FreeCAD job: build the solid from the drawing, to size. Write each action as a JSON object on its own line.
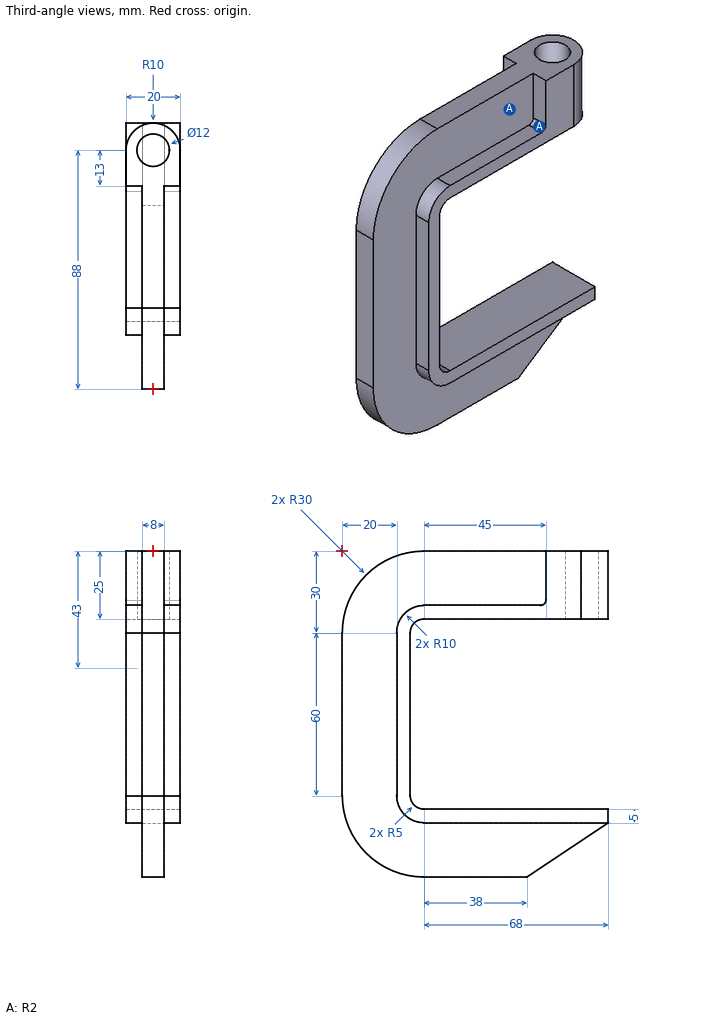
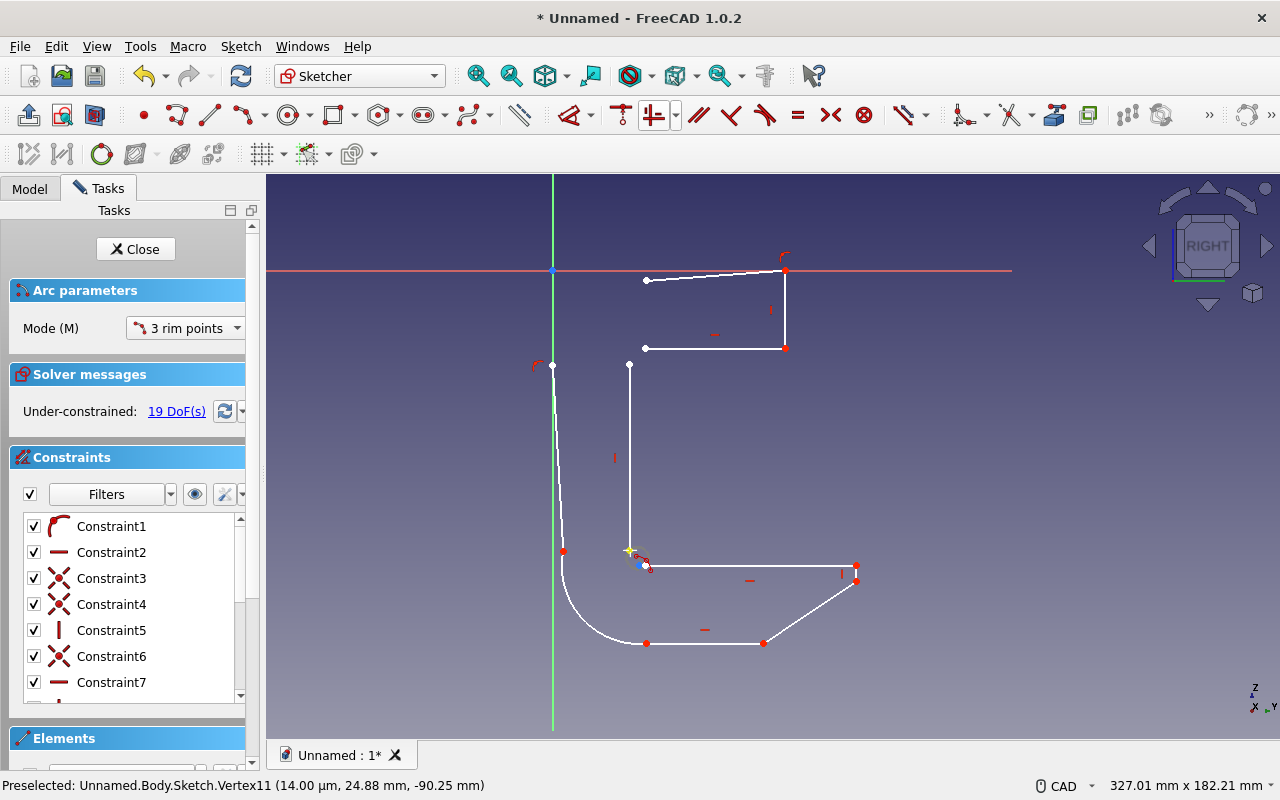
{"action": "scroll", "coordinate": [635, 561], "scroll_direction": "up", "scroll_amount": 7}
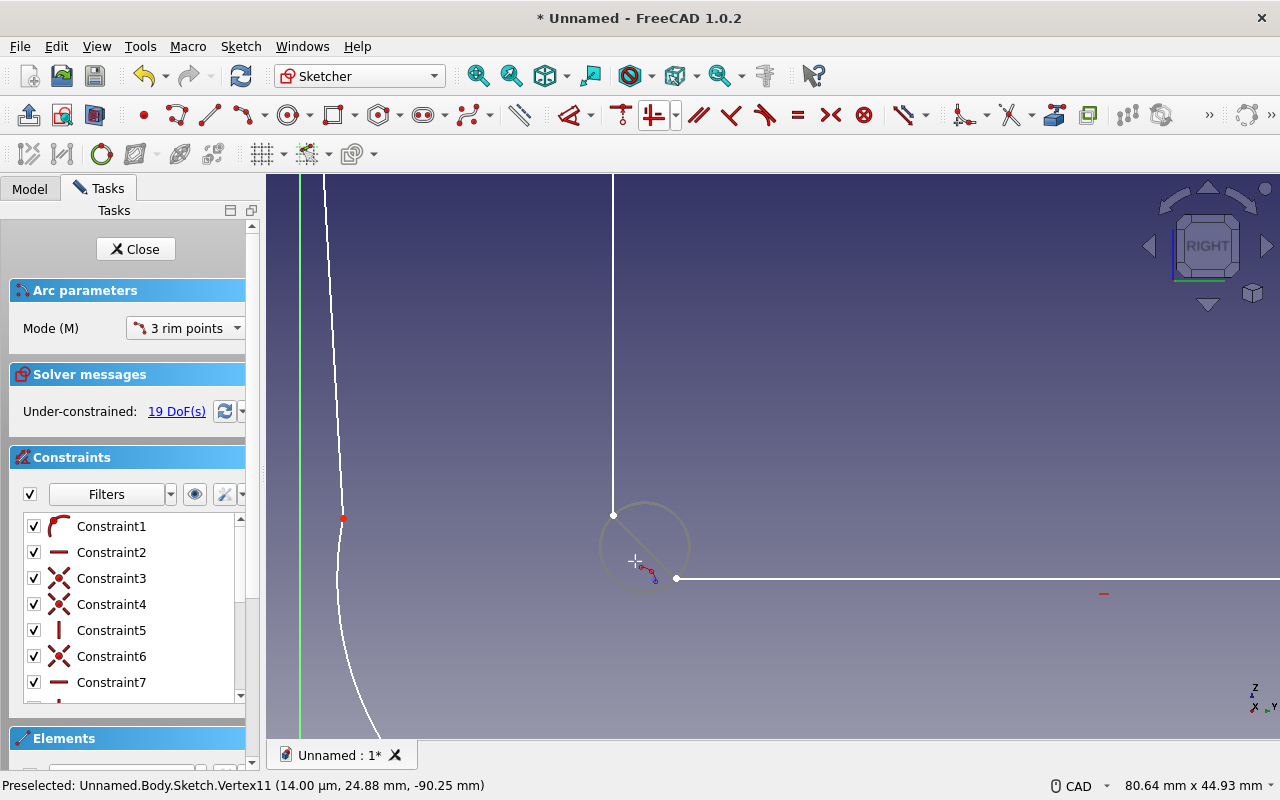
{"action": "left_click", "coordinate": [633, 557]}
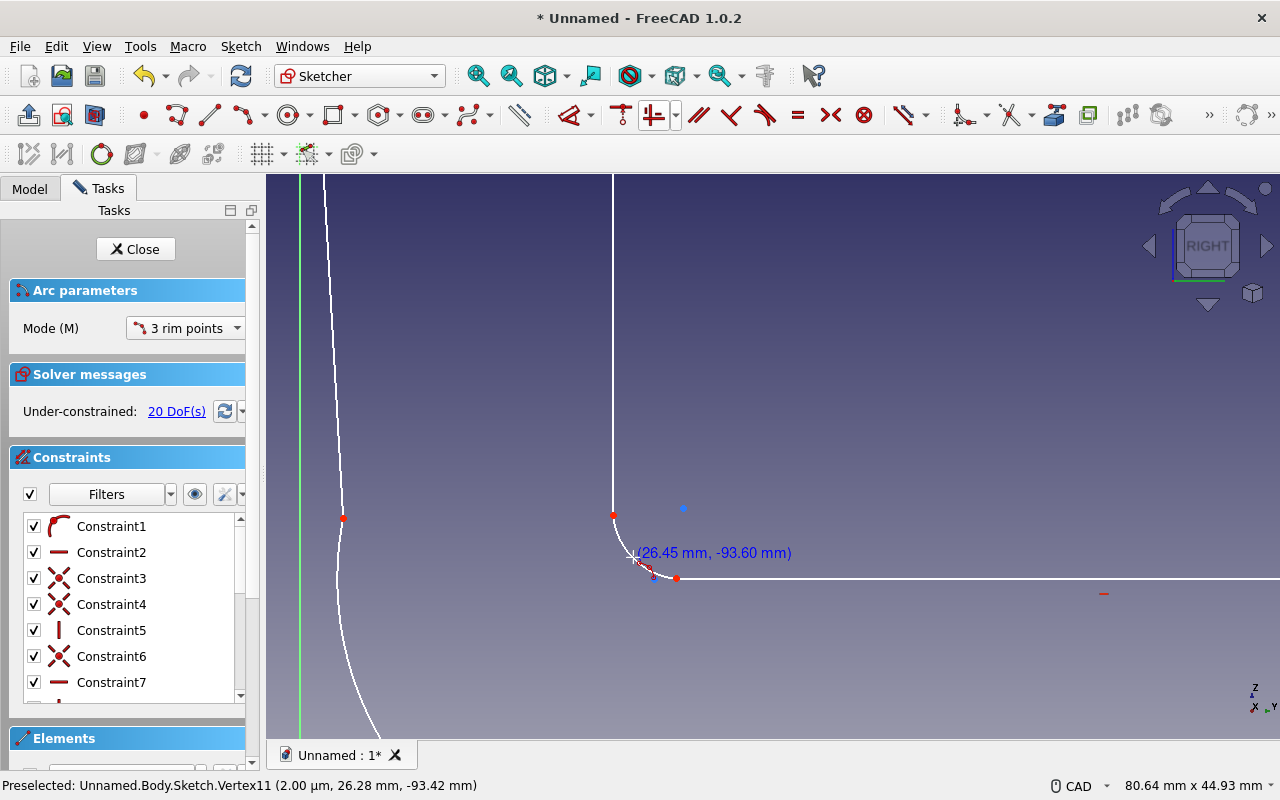
{"action": "scroll", "coordinate": [635, 562], "scroll_direction": "down", "scroll_amount": 7}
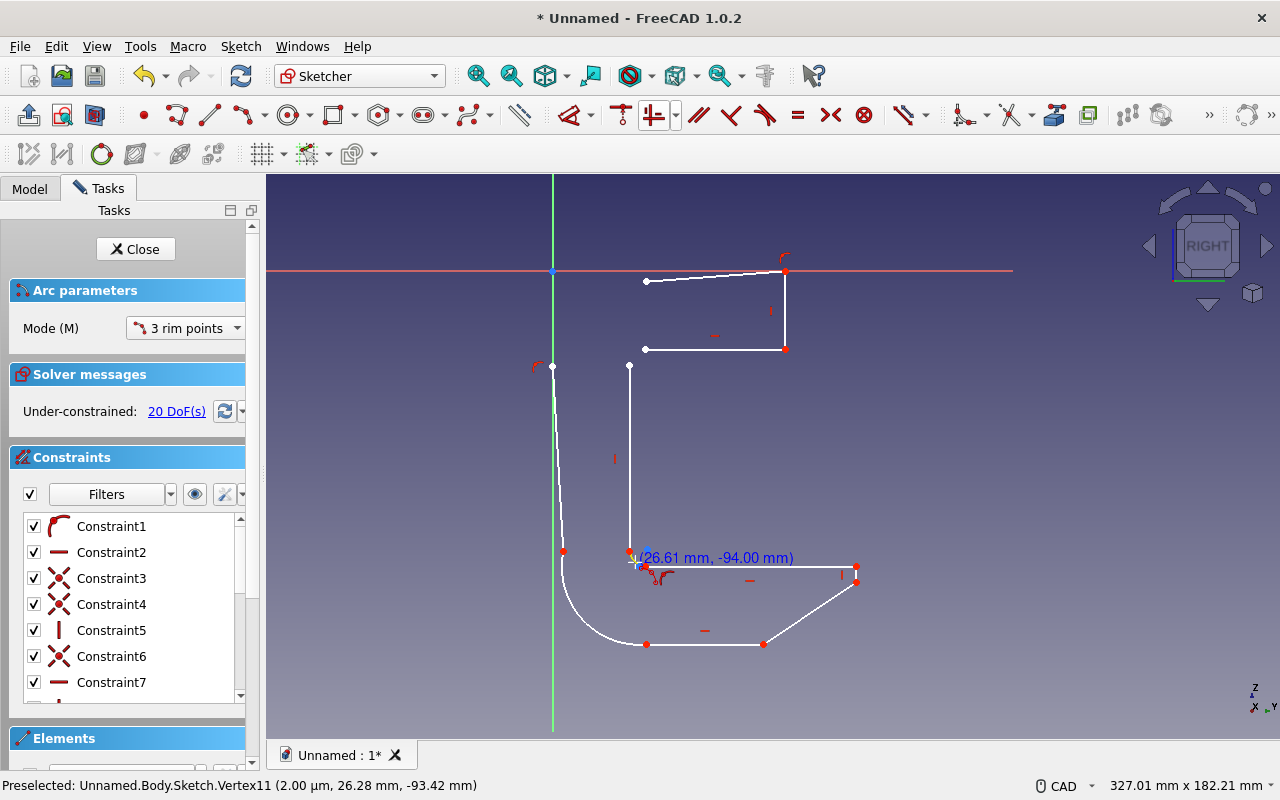
{"action": "left_click", "coordinate": [630, 365]}
{"action": "left_click", "coordinate": [645, 350]}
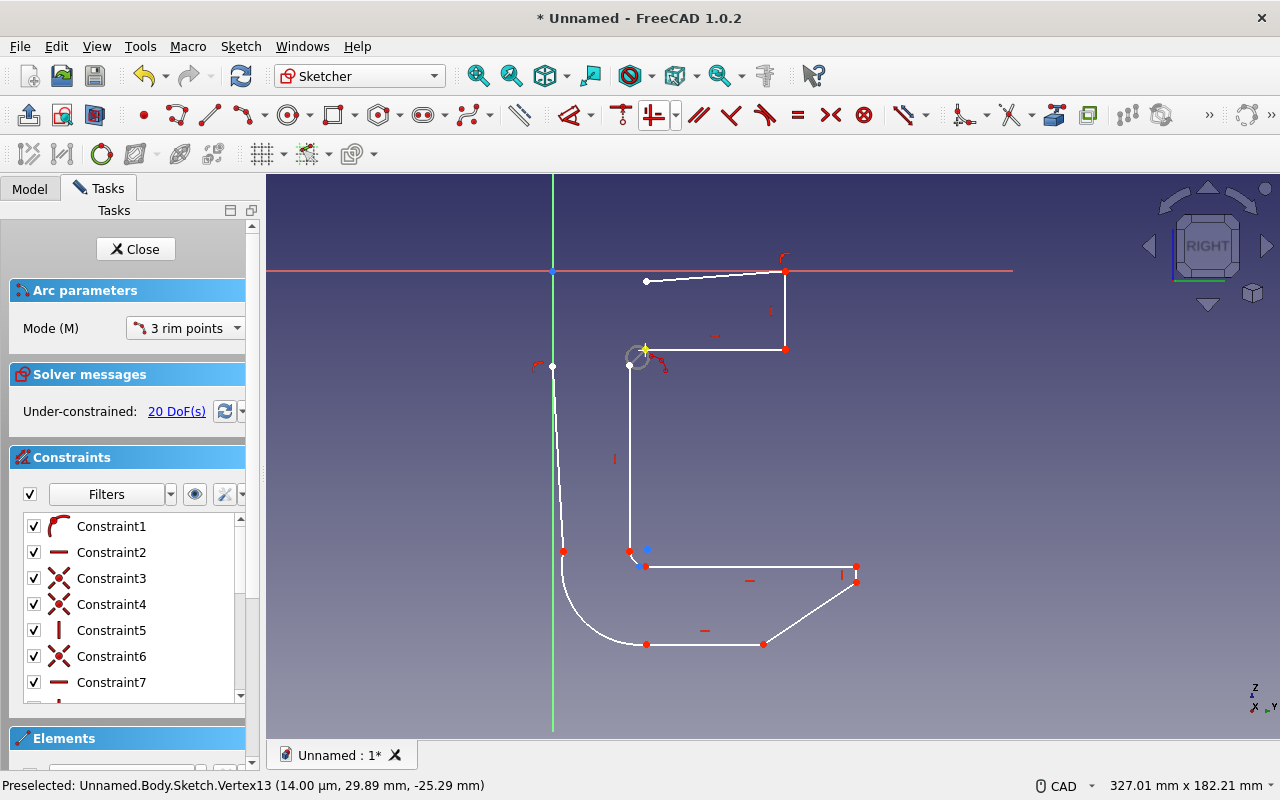
{"action": "scroll", "coordinate": [635, 353], "scroll_direction": "up", "scroll_amount": 7}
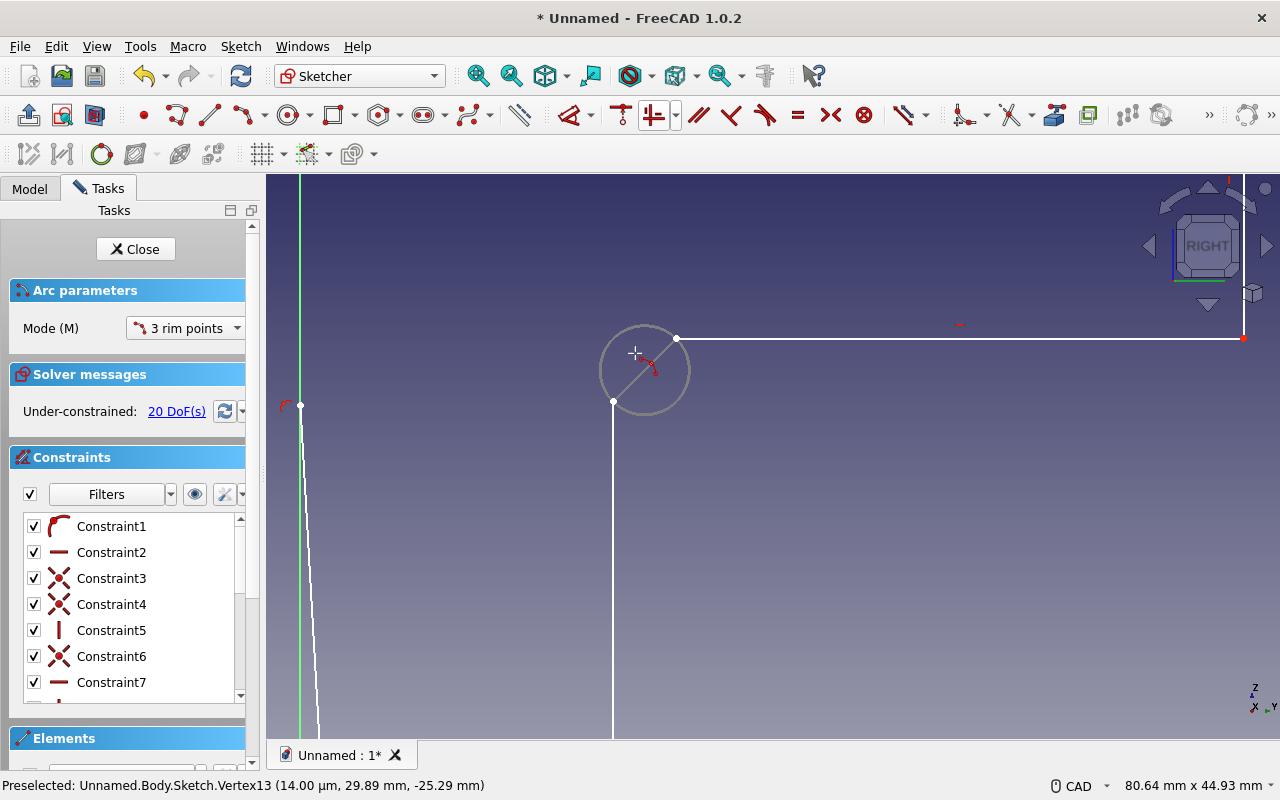
{"action": "left_click", "coordinate": [633, 353]}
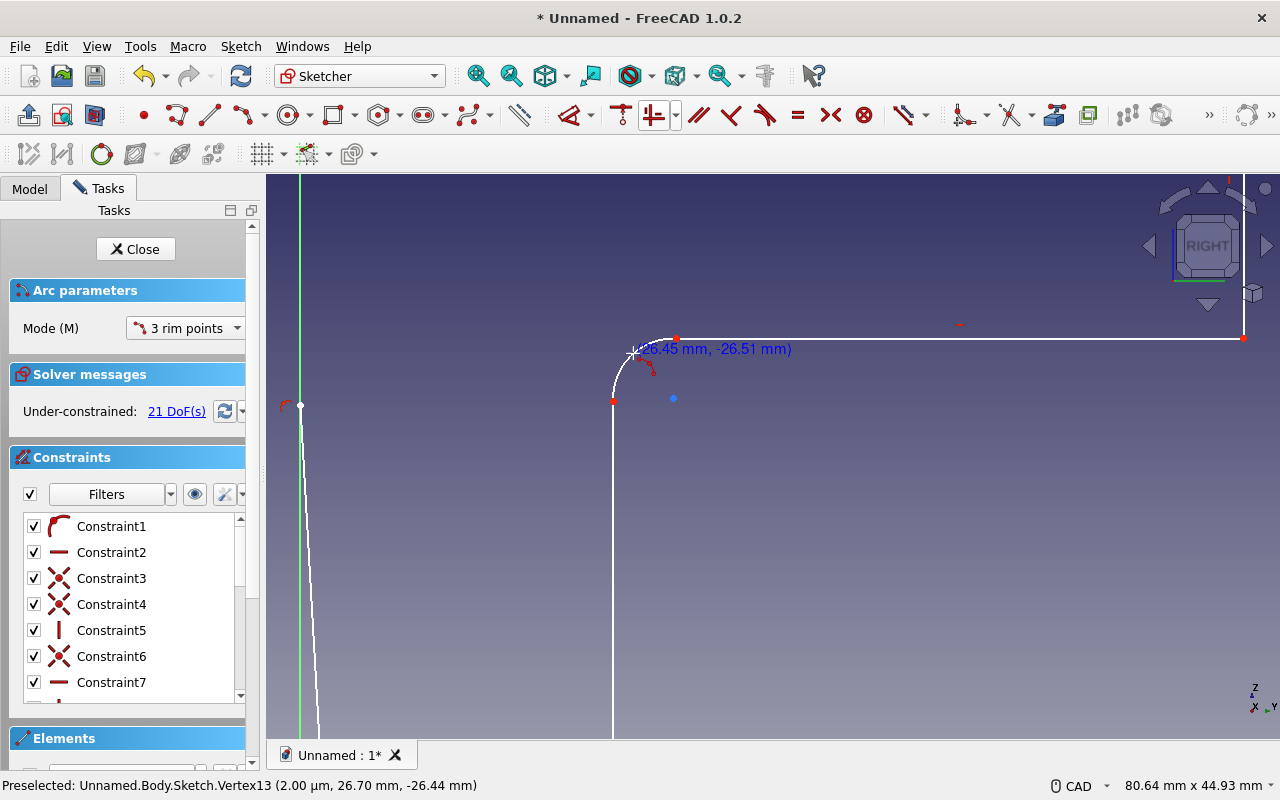
{"action": "scroll", "coordinate": [635, 352], "scroll_direction": "down", "scroll_amount": 7}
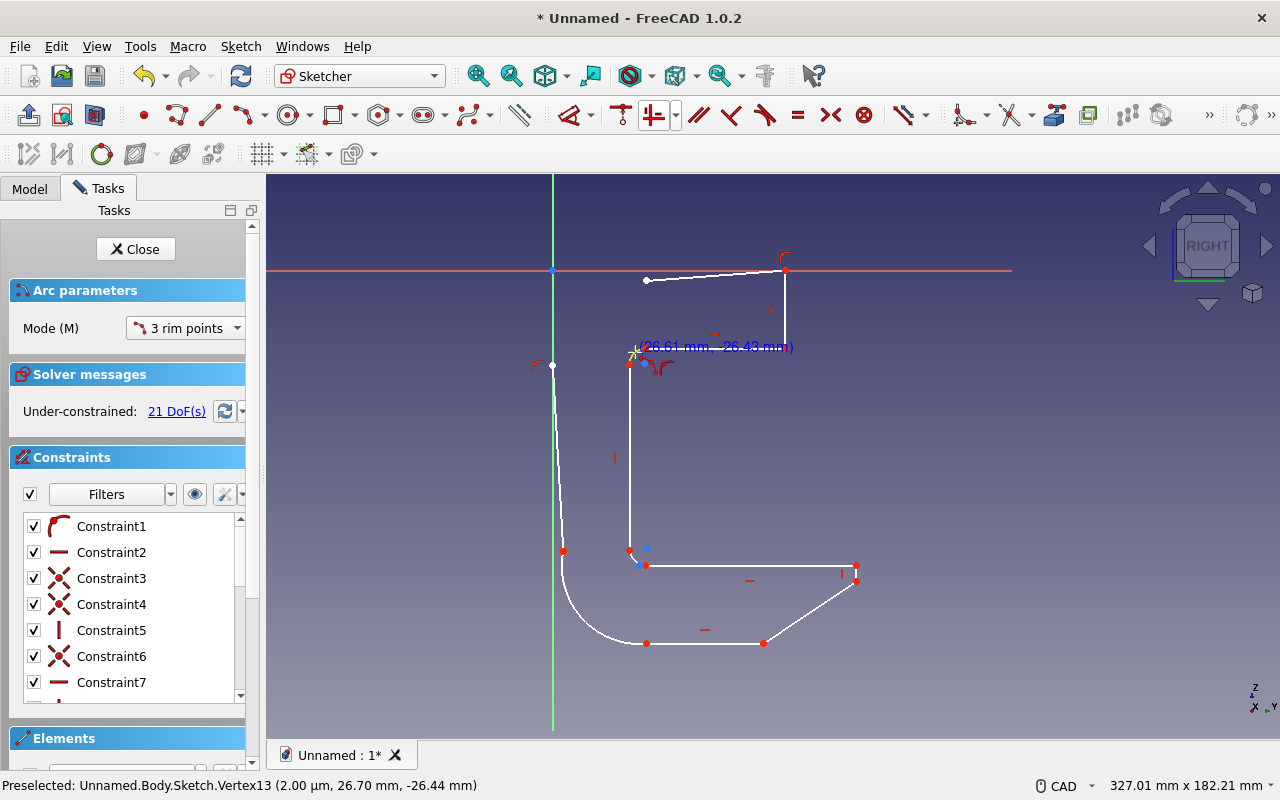
{"action": "left_click", "coordinate": [646, 281]}
{"action": "left_click", "coordinate": [553, 365]}
{"action": "left_click", "coordinate": [580, 298]}
{"action": "key", "text": "Escape"}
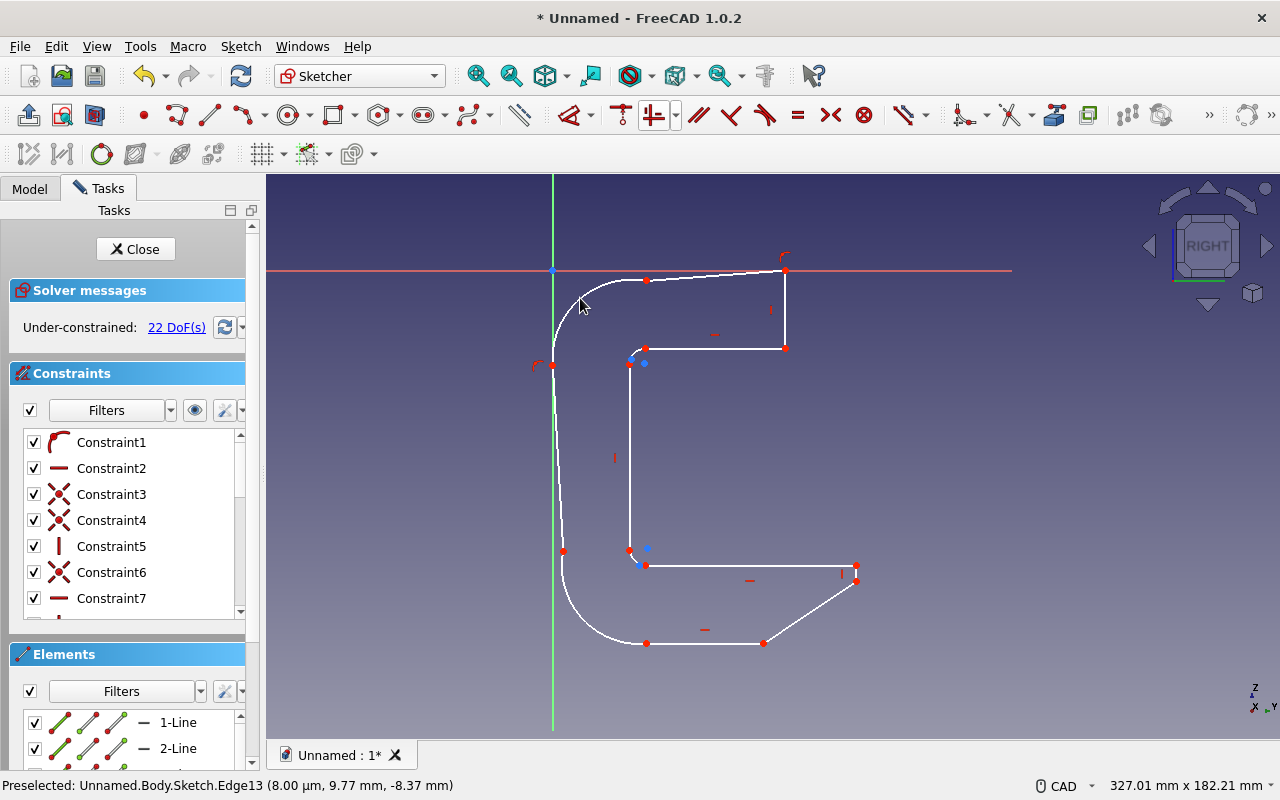
{"action": "left_click", "coordinate": [556, 421]}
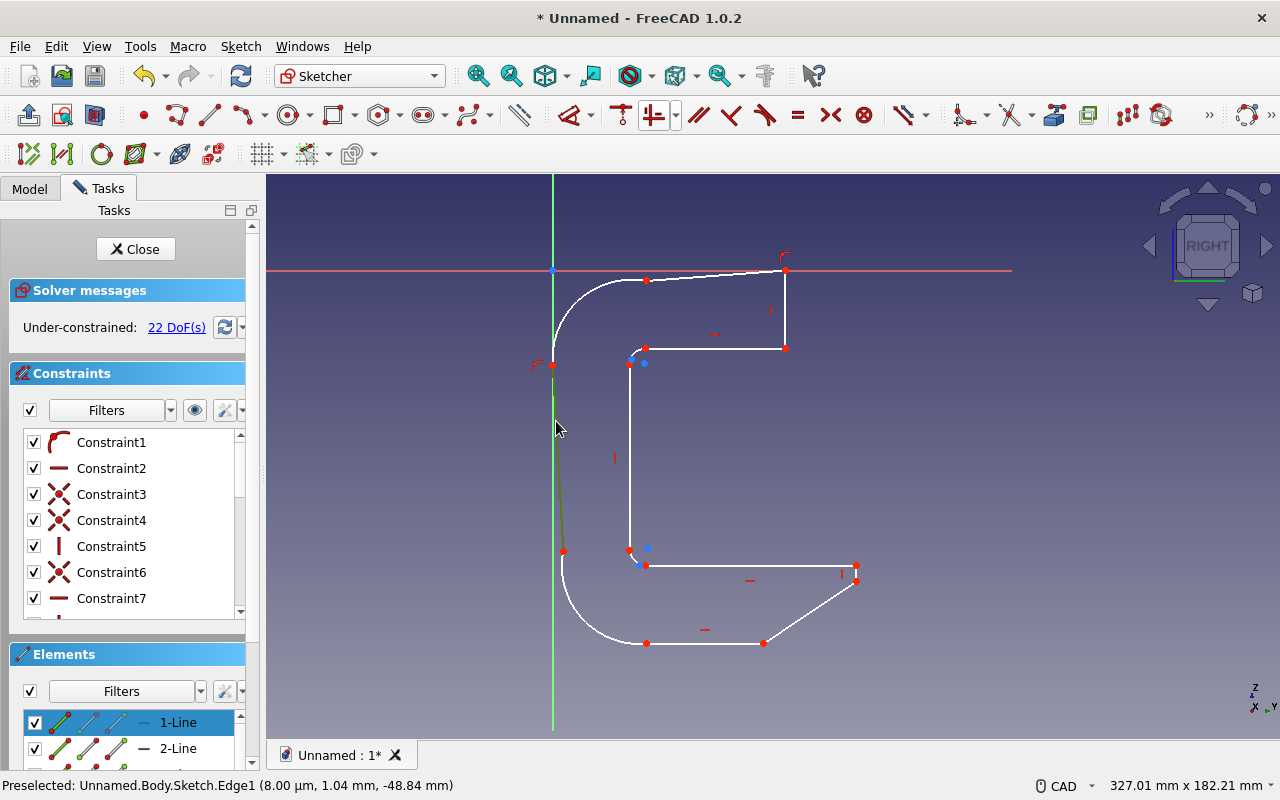
{"action": "left_click", "coordinate": [567, 594]}